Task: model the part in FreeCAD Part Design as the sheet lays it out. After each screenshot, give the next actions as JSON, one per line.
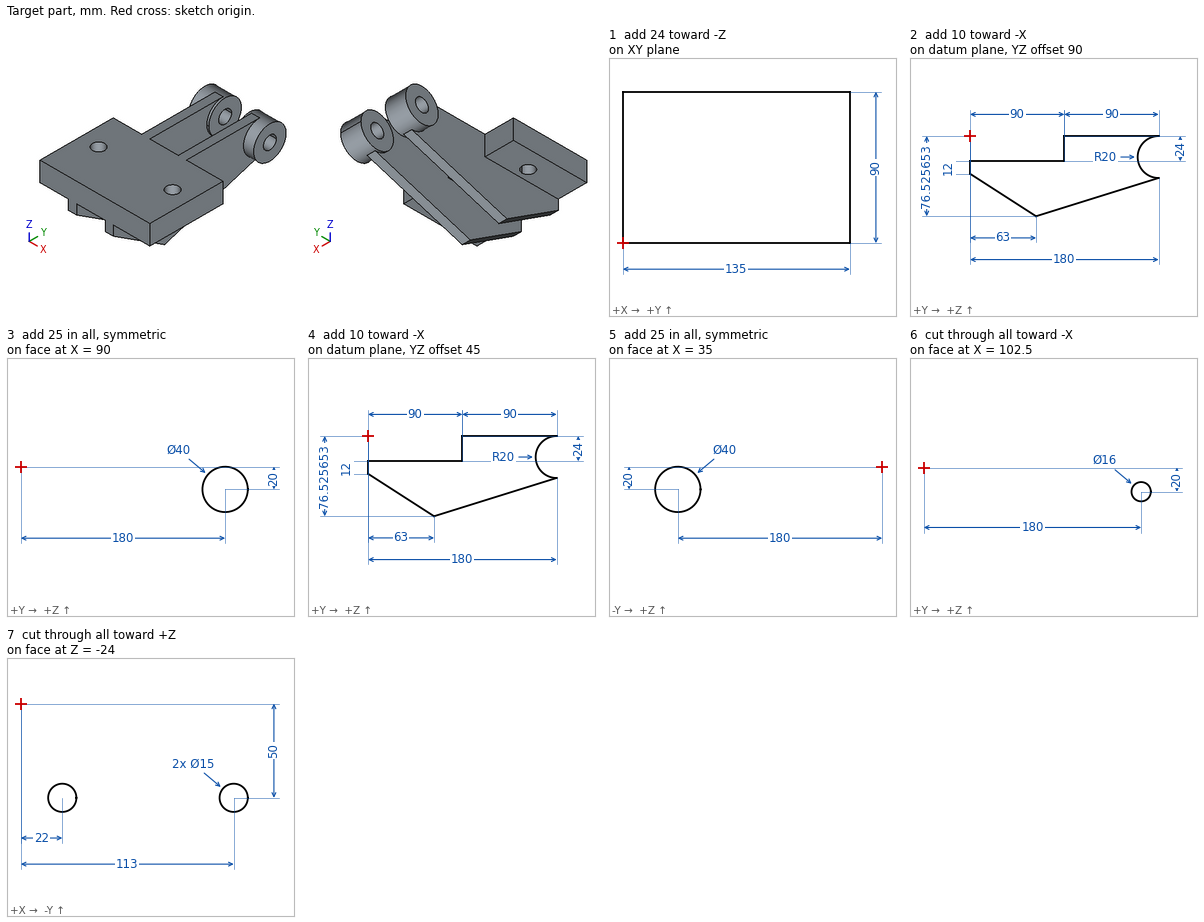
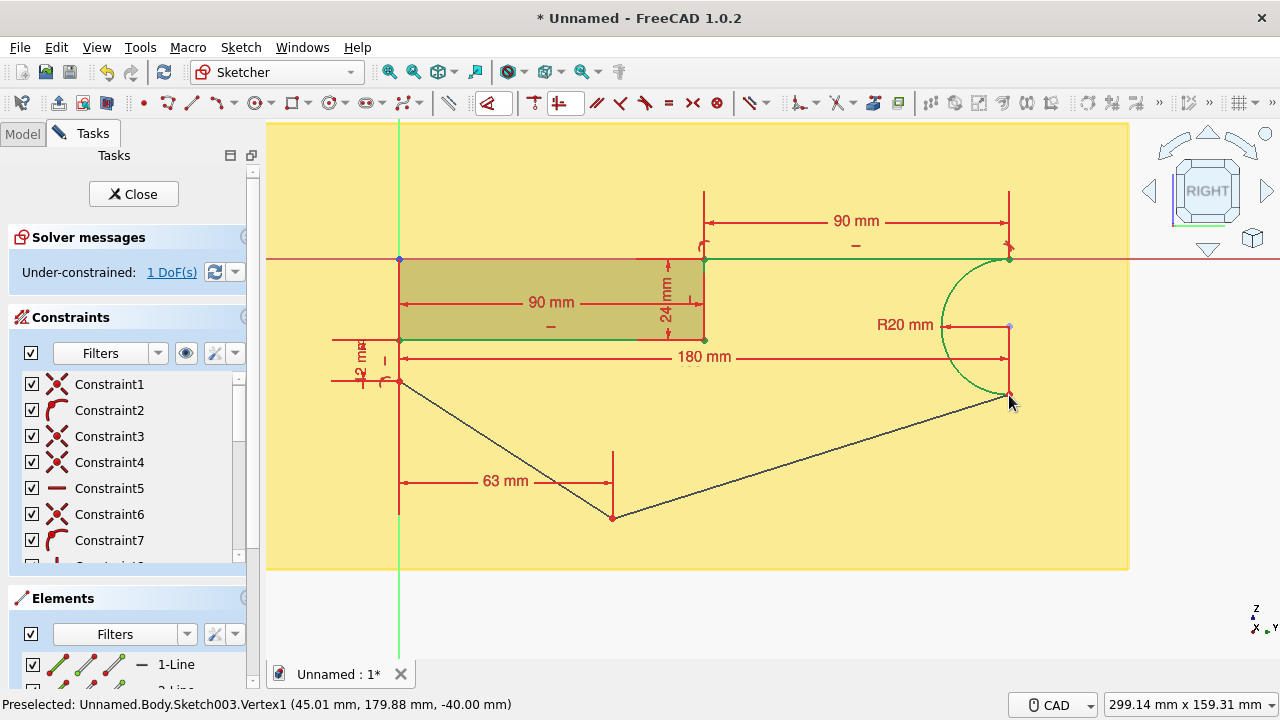
{"action": "left_click", "coordinate": [613, 519]}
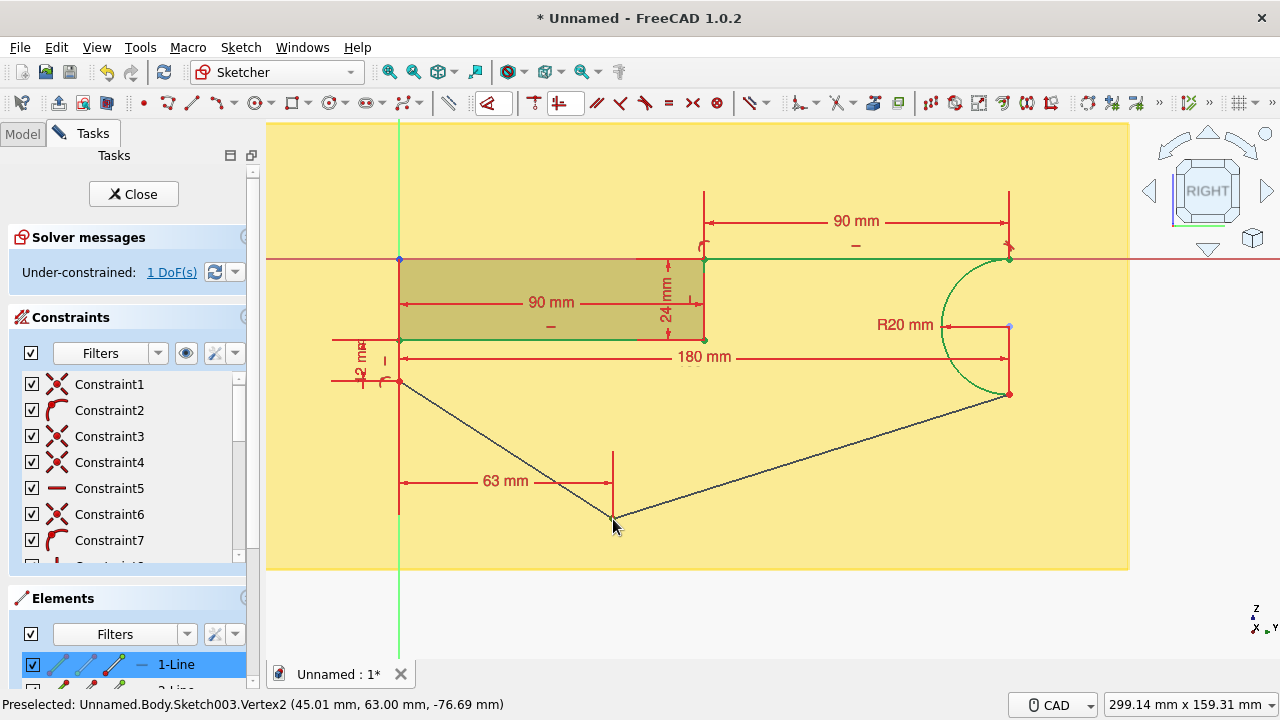
{"action": "key", "text": "i"}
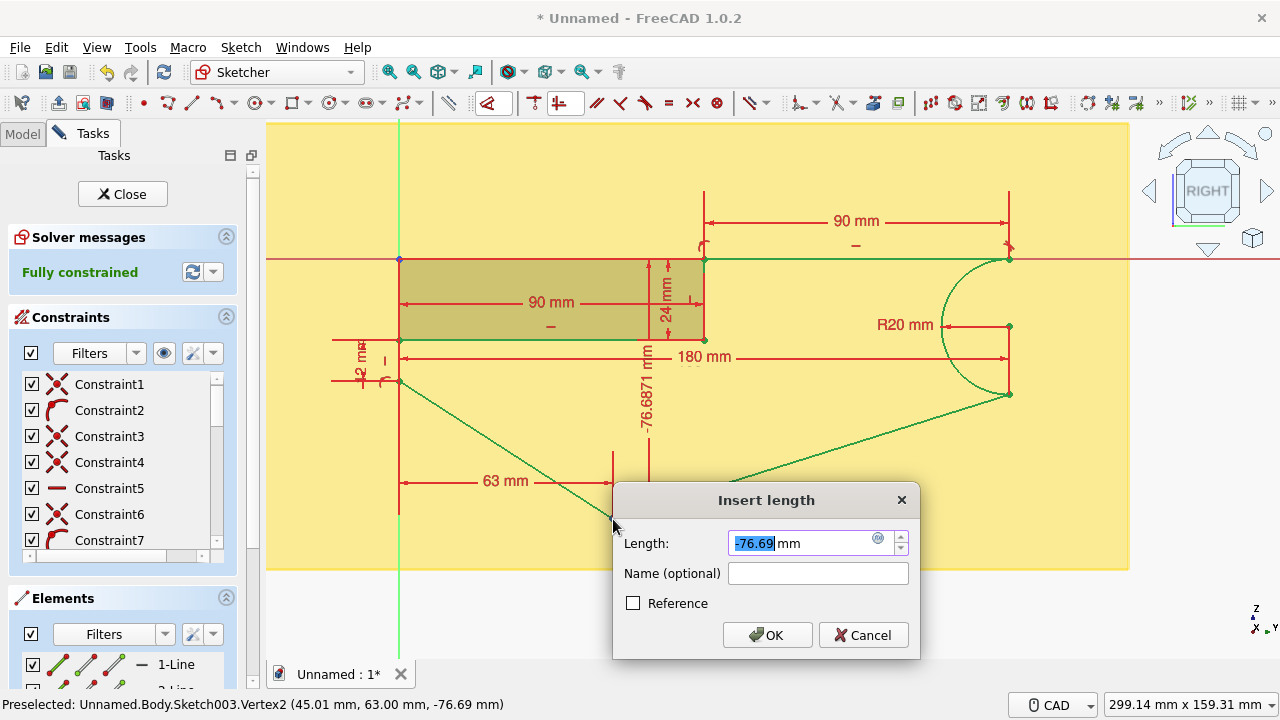
{"action": "type", "text": "-76.525653"}
{"action": "key", "text": "Return"}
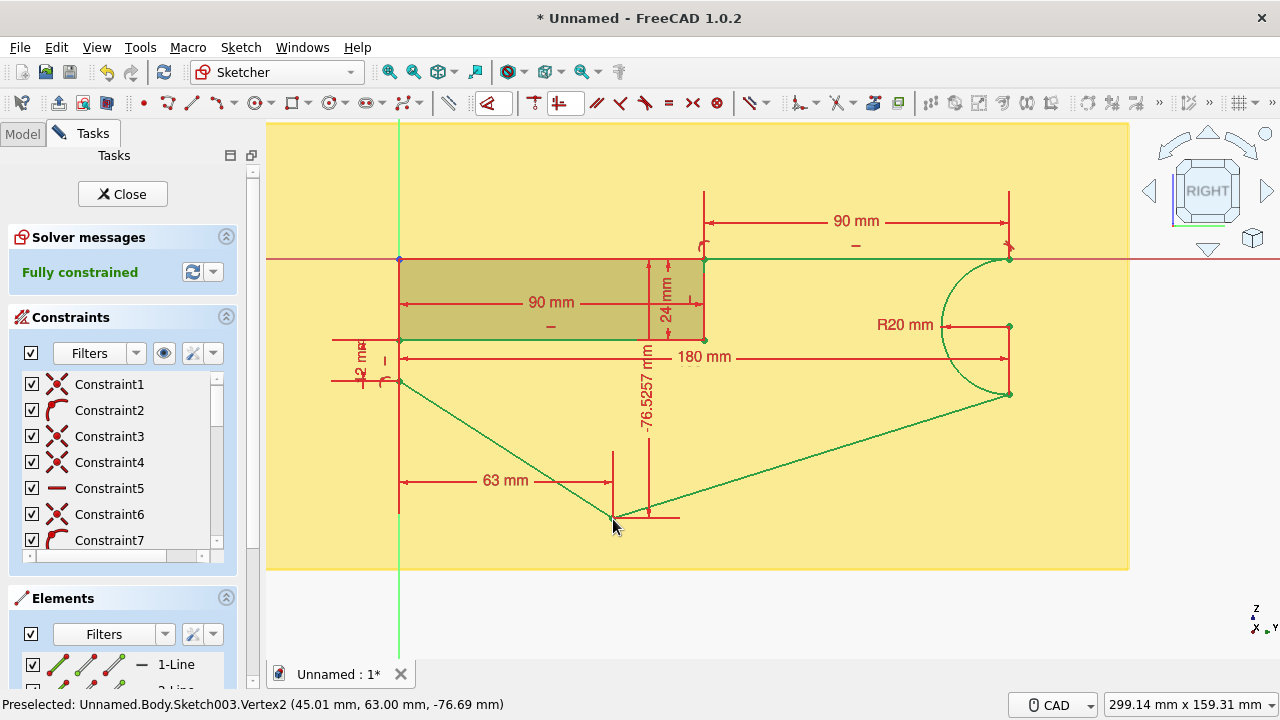
{"action": "left_click", "coordinate": [123, 194]}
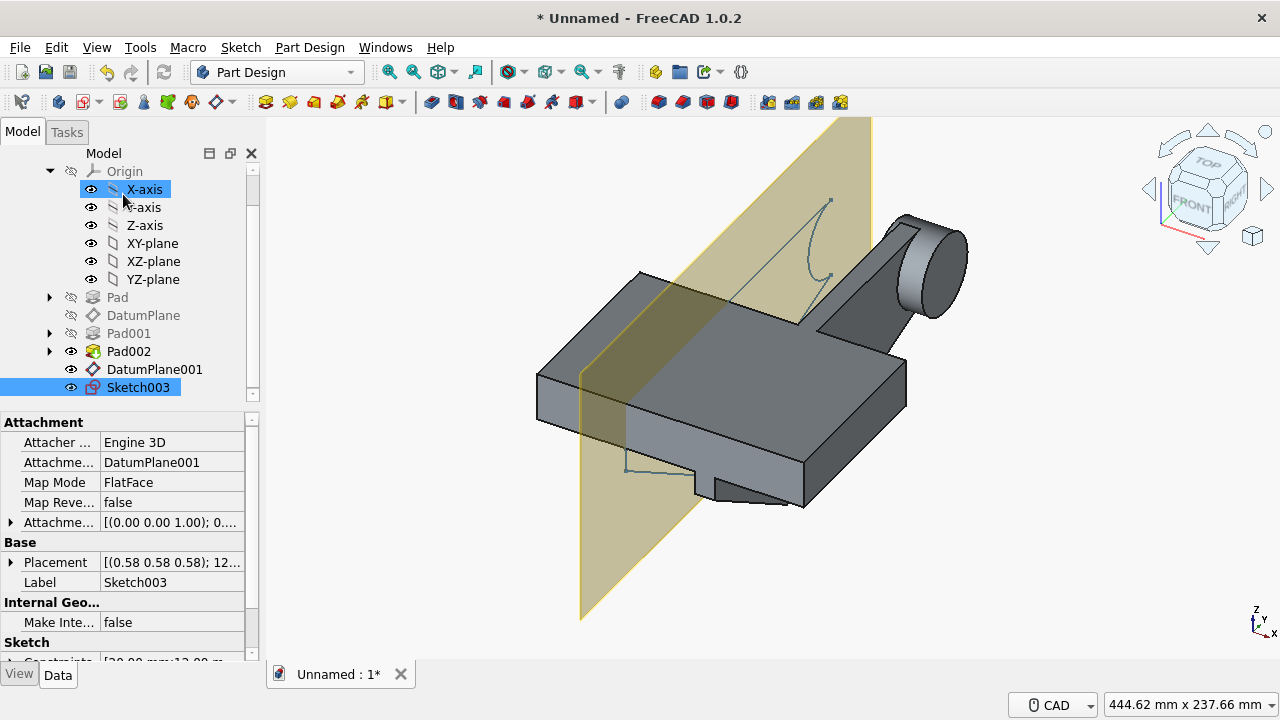
{"action": "left_click", "coordinate": [266, 102]}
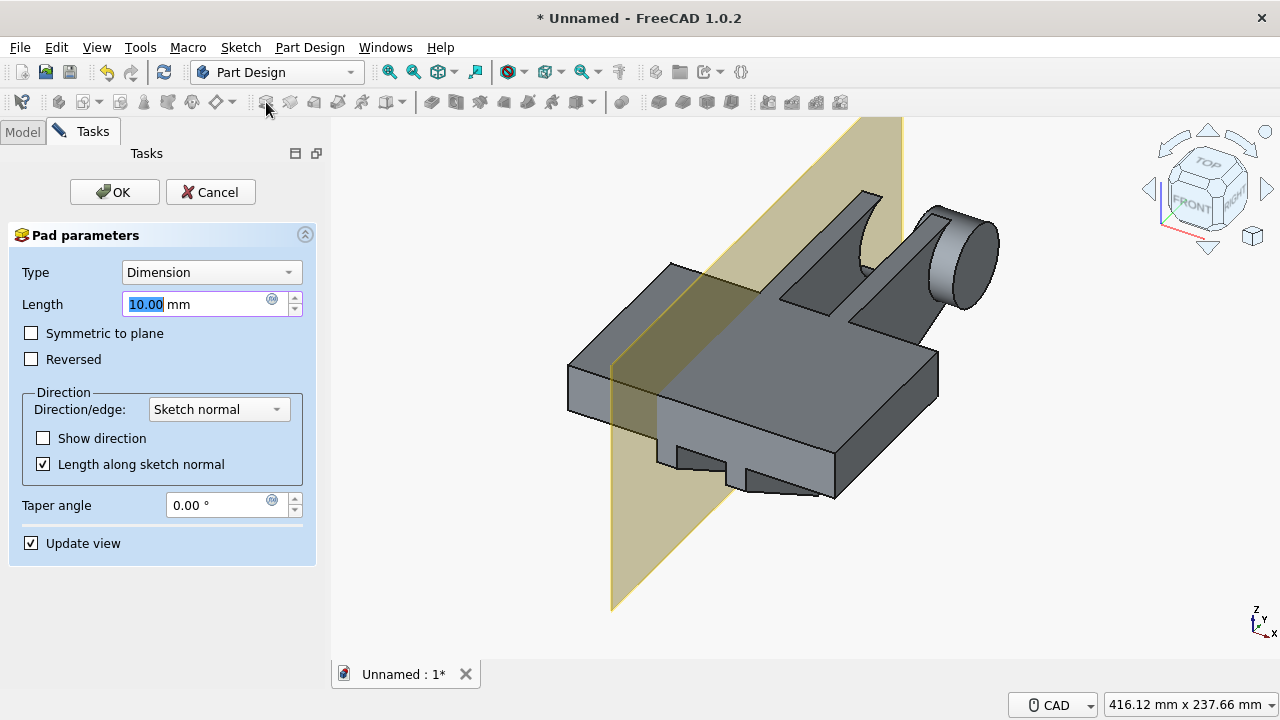
{"action": "type", "text": "10"}
{"action": "key", "text": "Tab"}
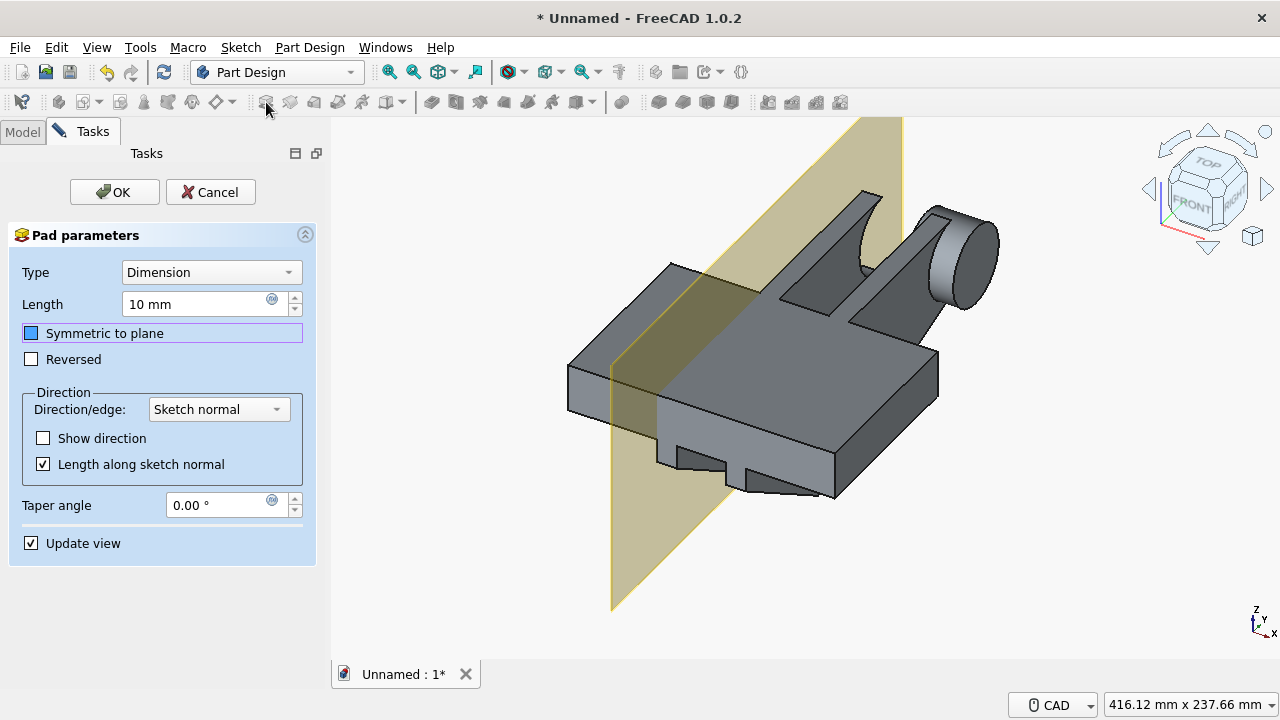
{"action": "left_click", "coordinate": [30, 359]}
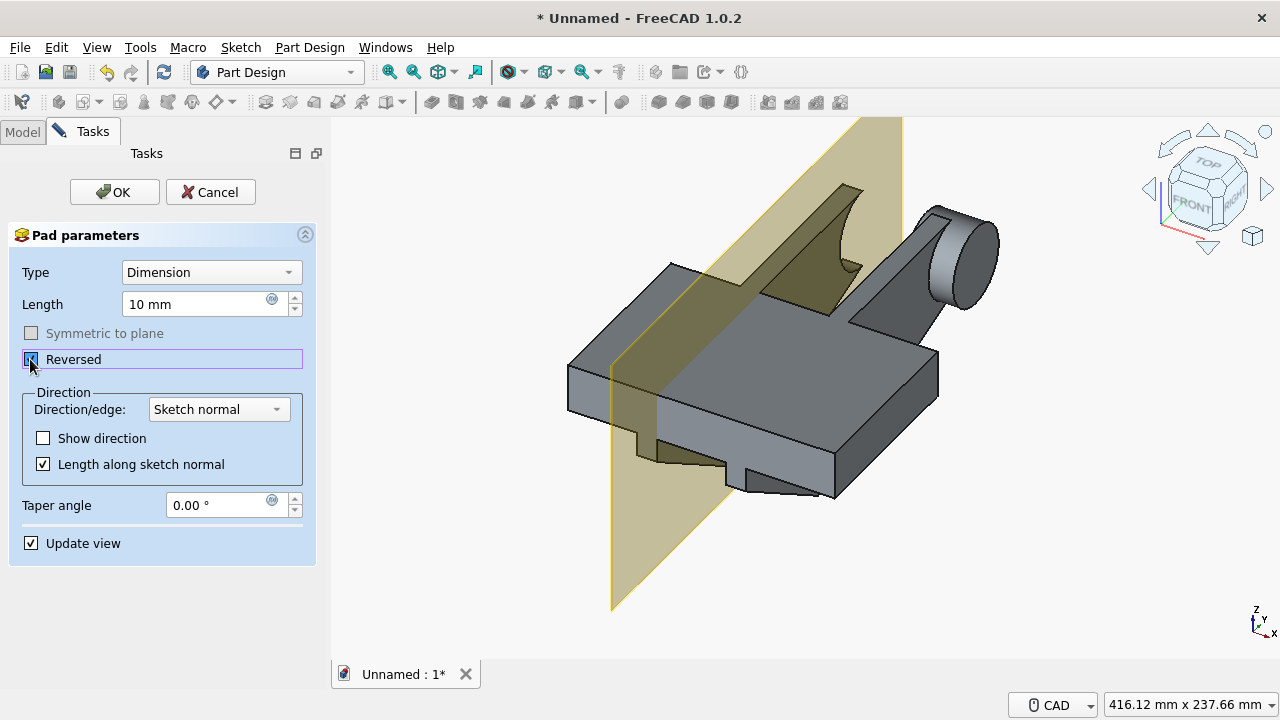
{"action": "left_click", "coordinate": [115, 192]}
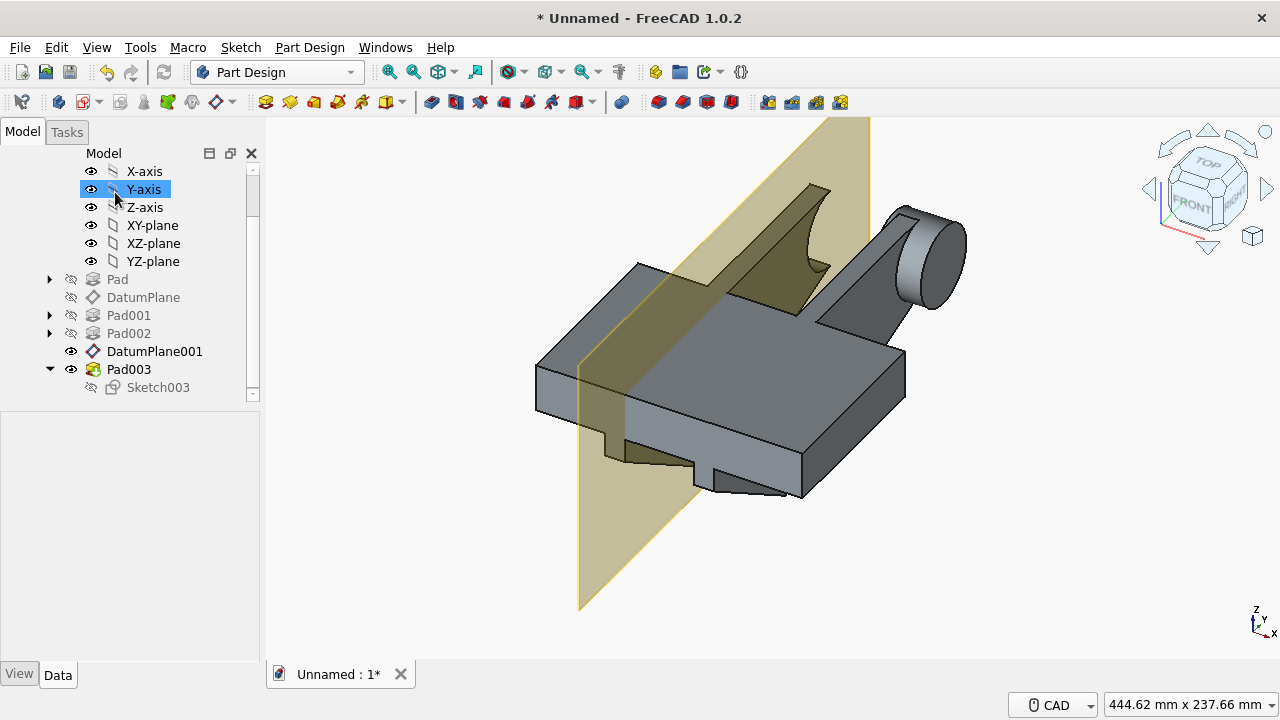
{"action": "left_click", "coordinate": [116, 351]}
{"action": "key", "text": "space"}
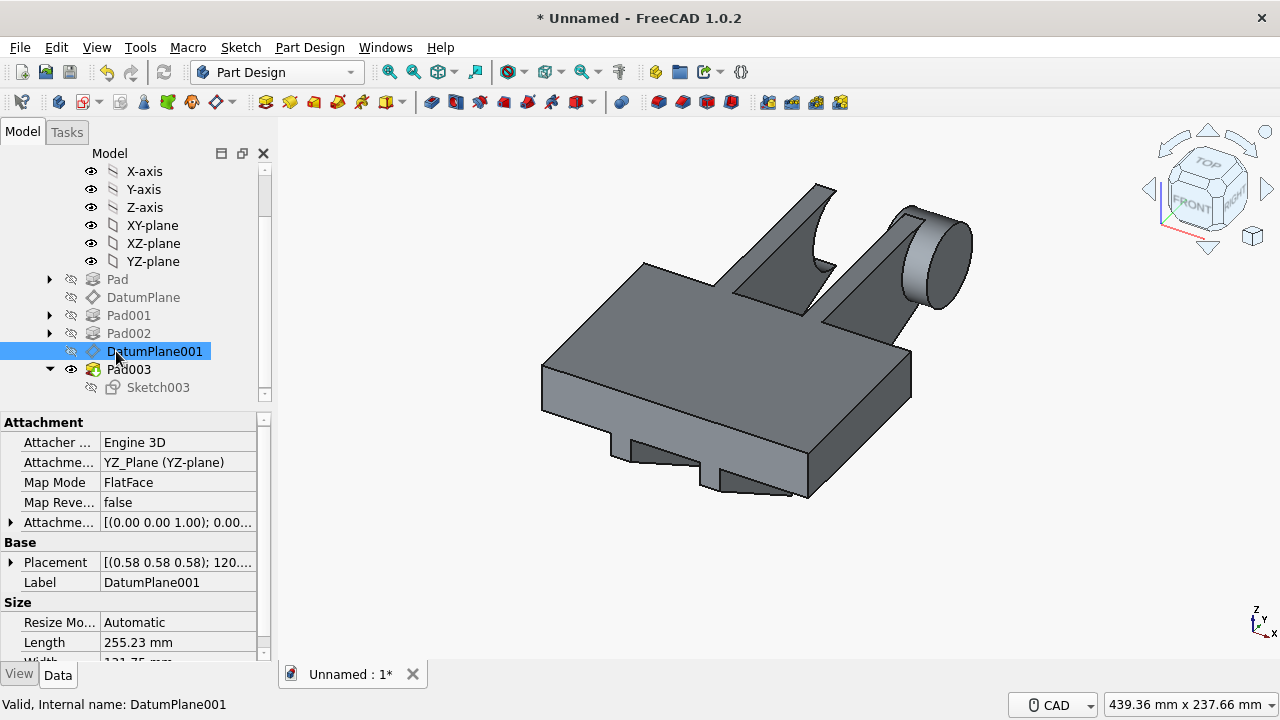
{"action": "key", "text": "6"}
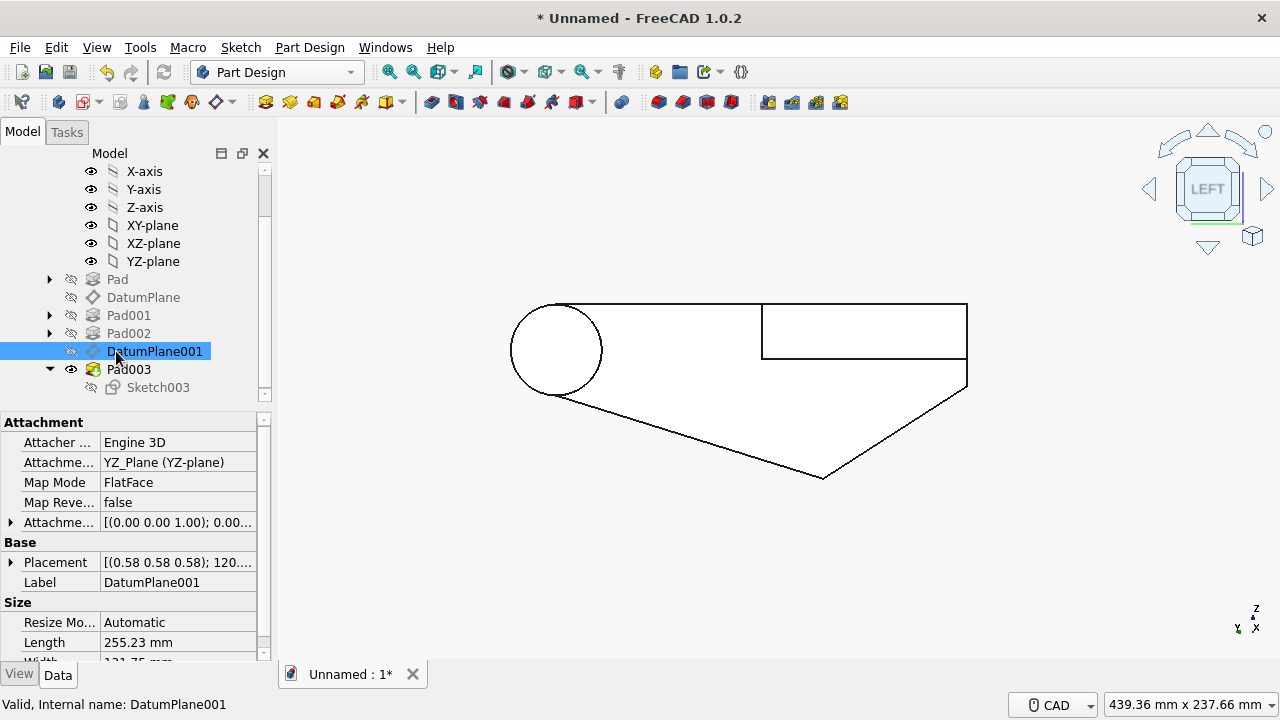
{"action": "left_click", "coordinate": [703, 366]}